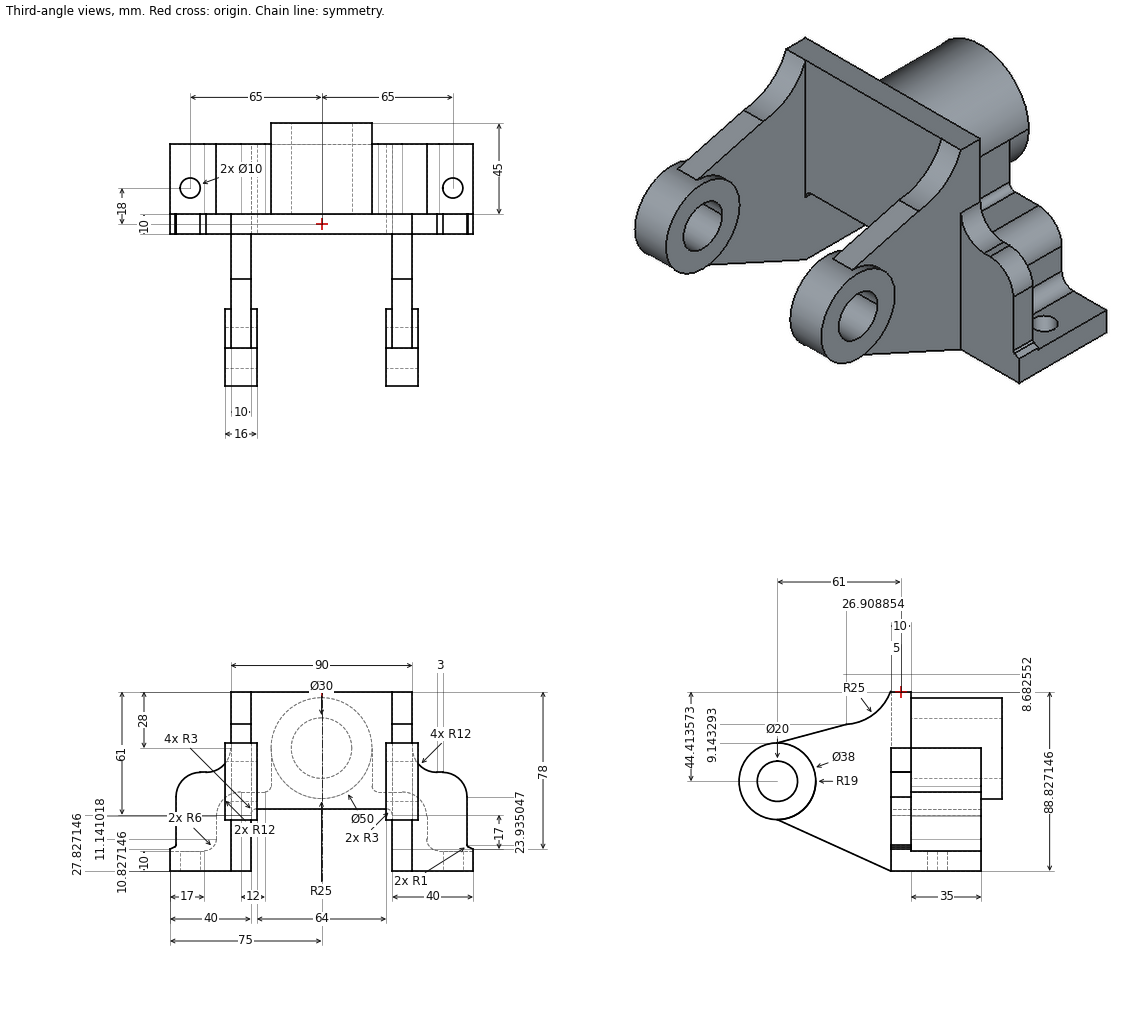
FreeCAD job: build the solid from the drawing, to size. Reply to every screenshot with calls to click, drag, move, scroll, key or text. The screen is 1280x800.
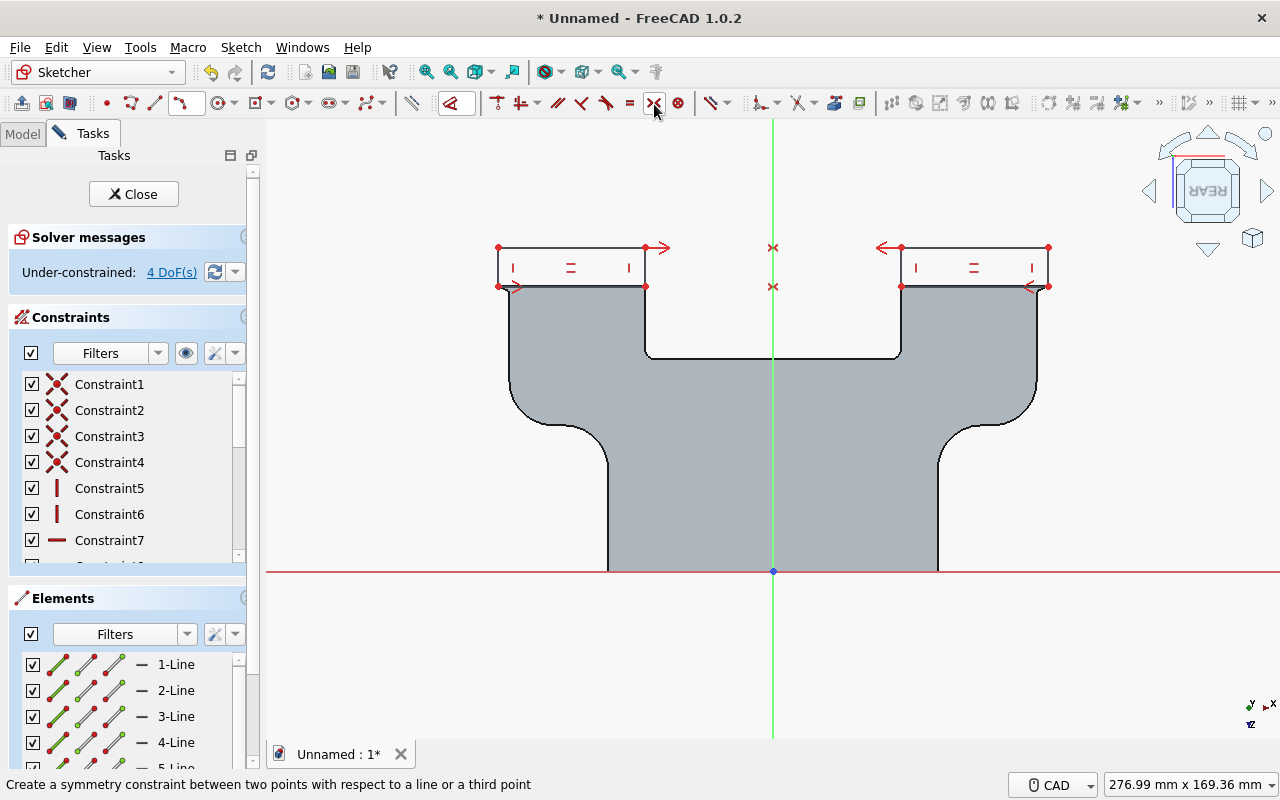
key(d)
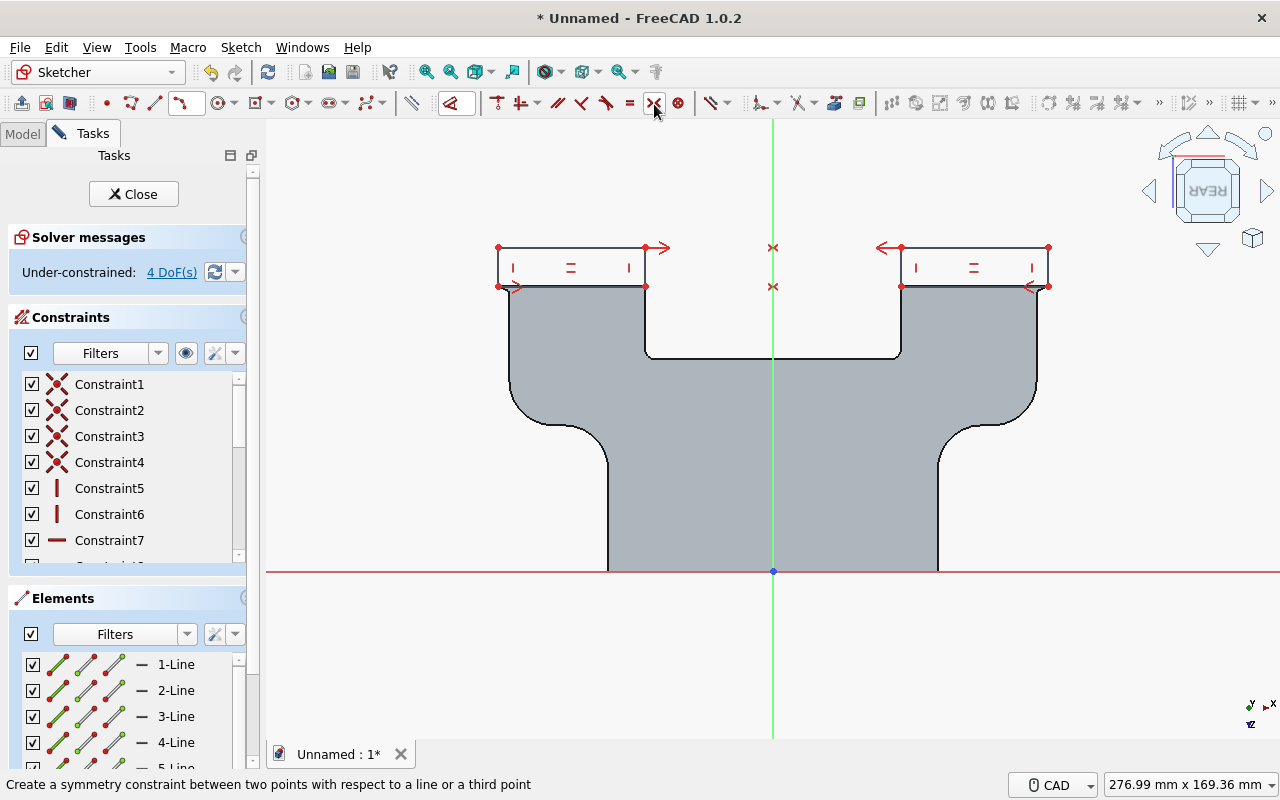
click(542, 287)
click(572, 321)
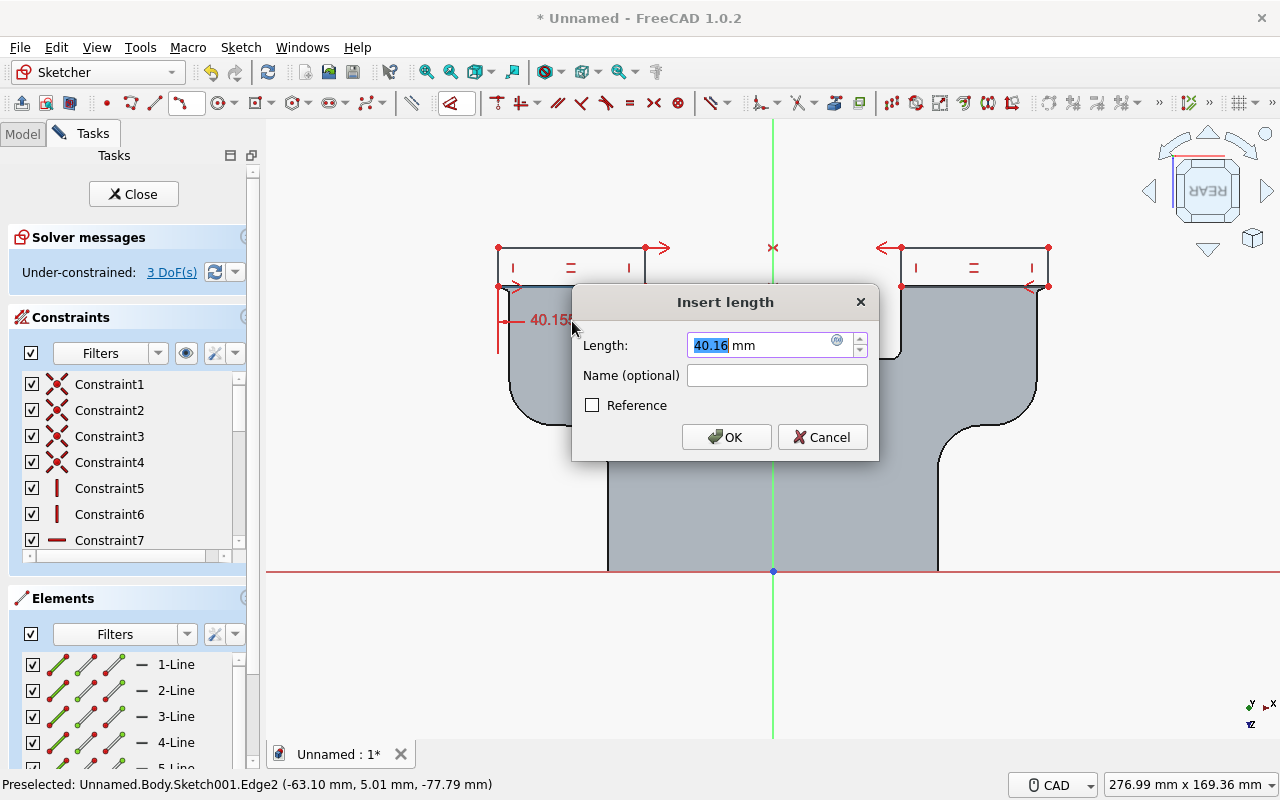
text(40)
key(Return)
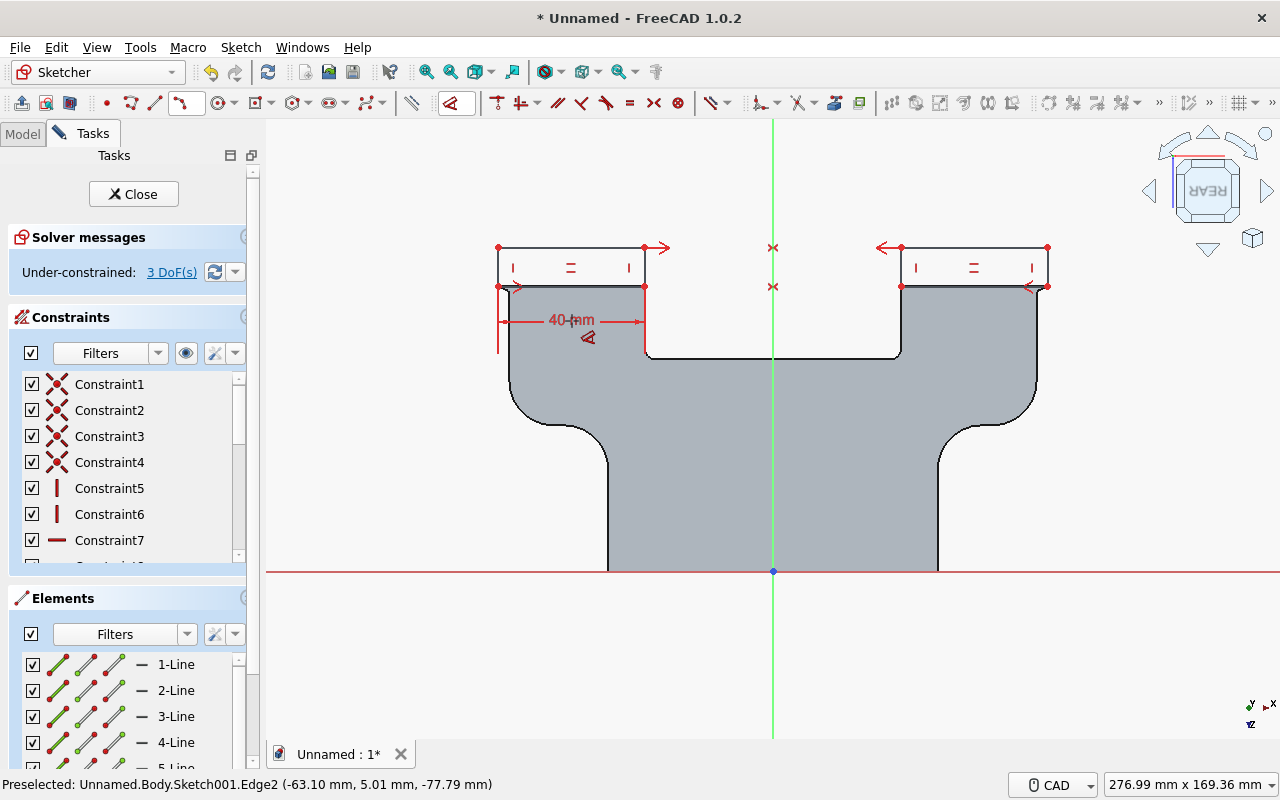
click(498, 248)
click(636, 606)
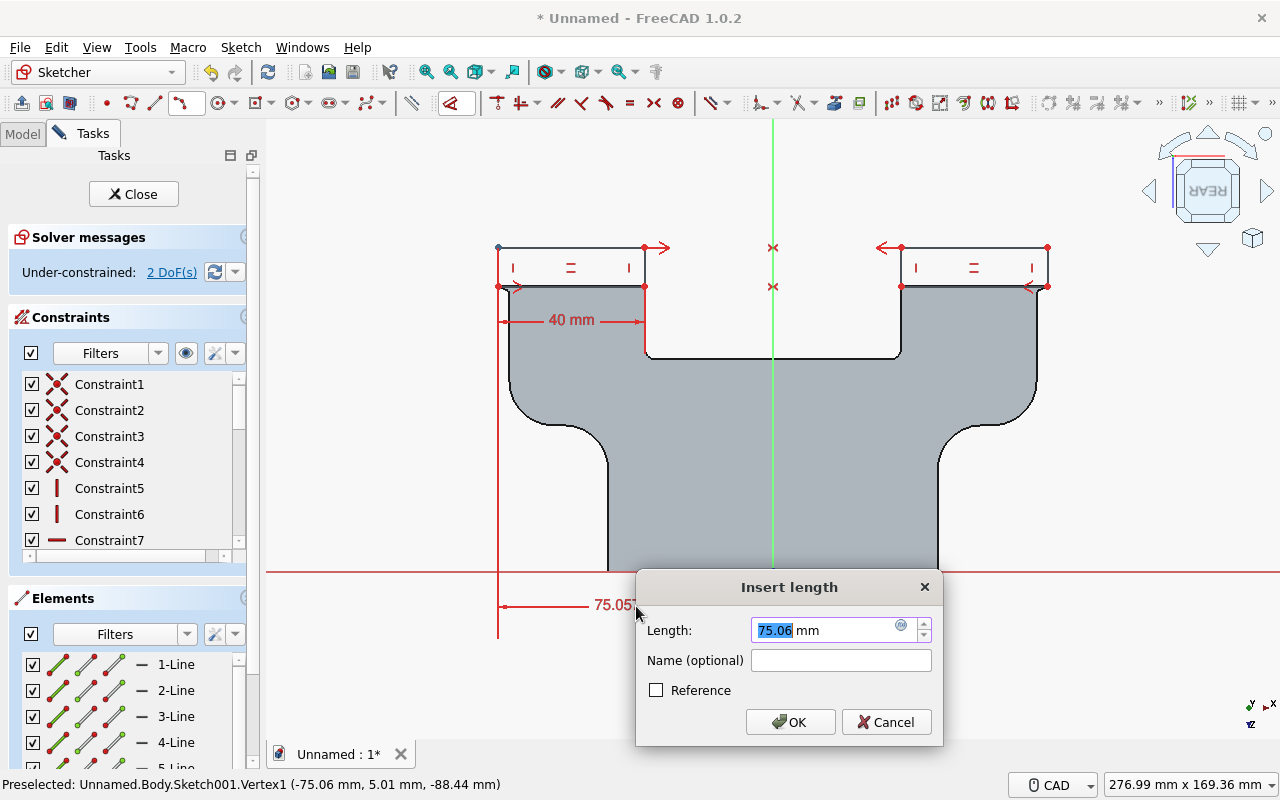
text(75)
key(Return)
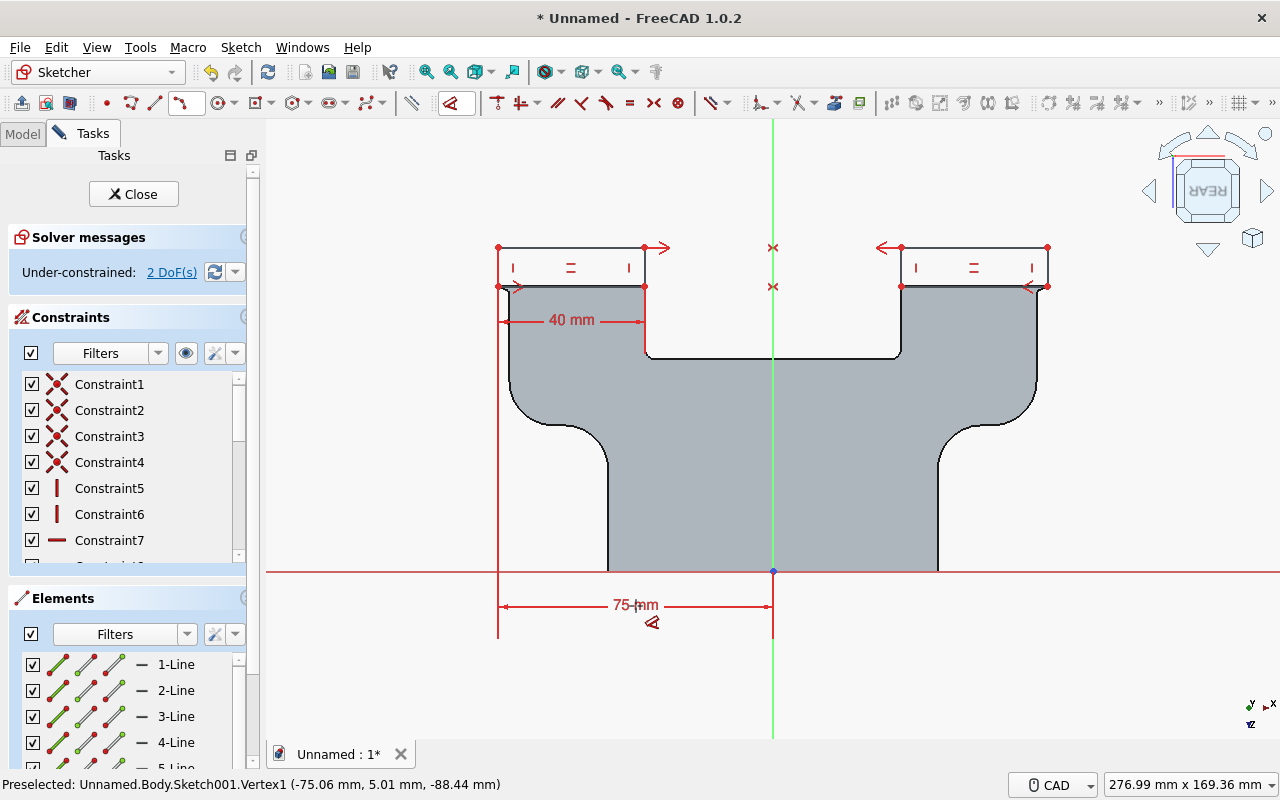
click(498, 287)
click(464, 429)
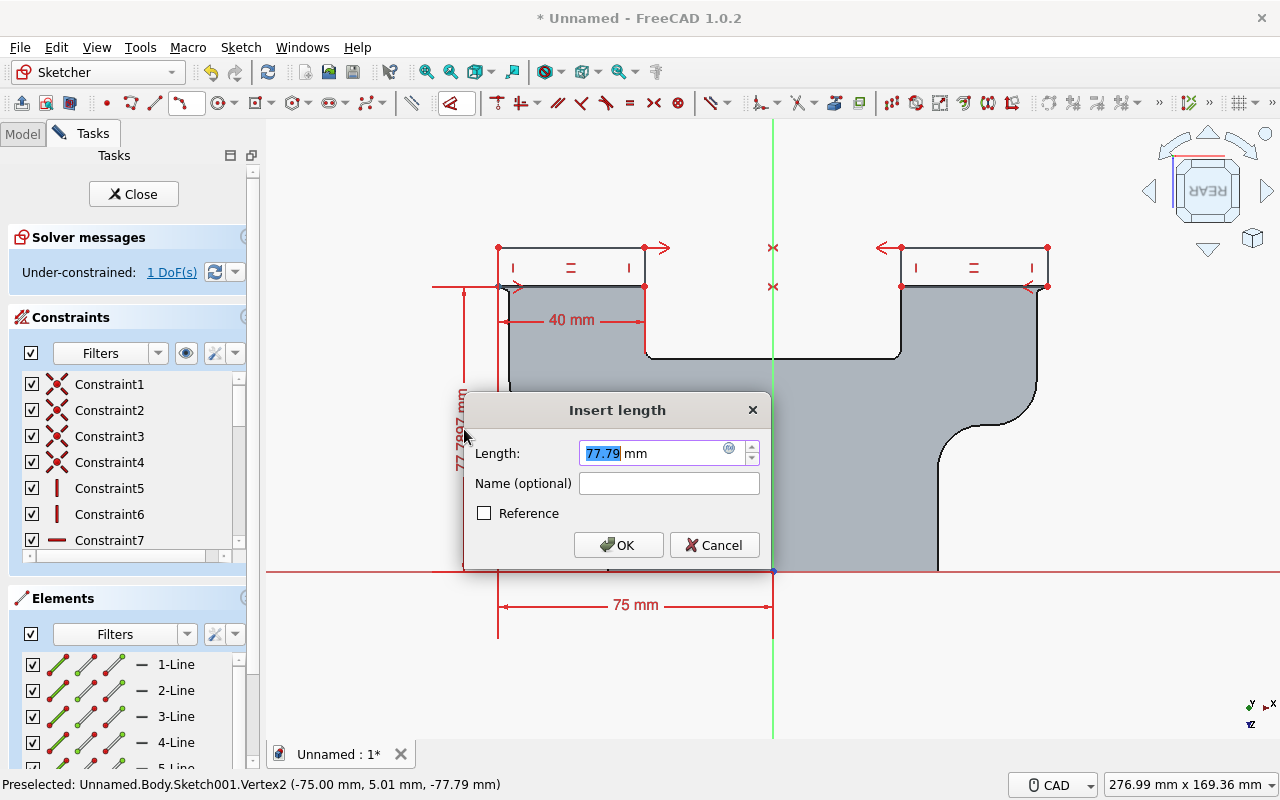
text(78)
key(Return)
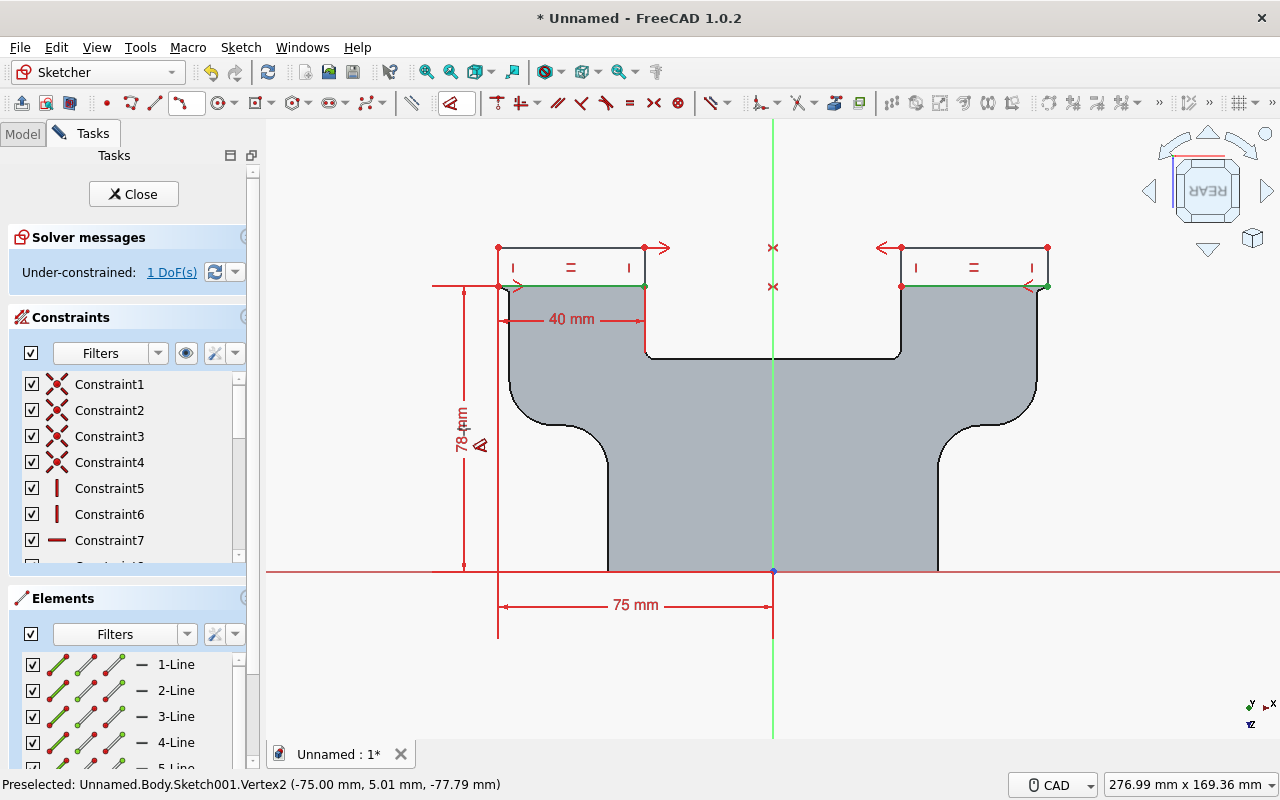
click(498, 259)
click(464, 267)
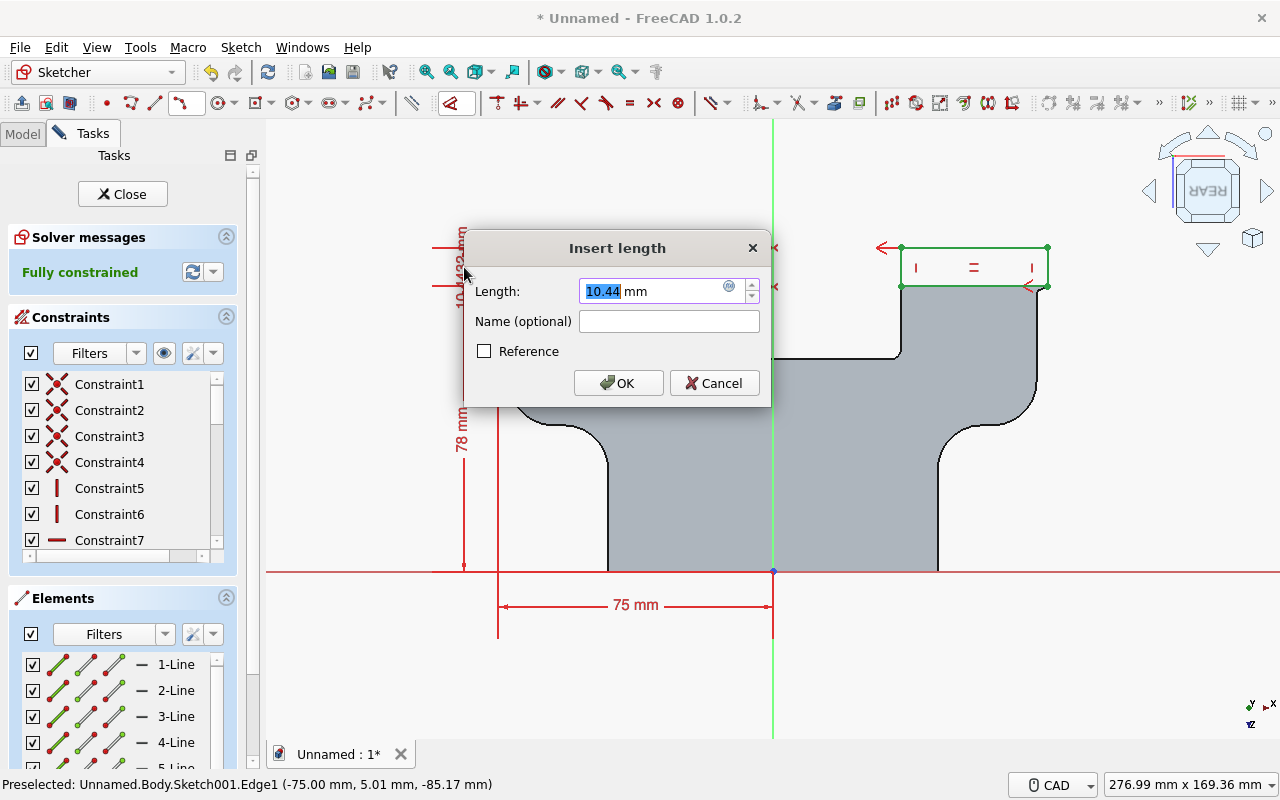
text(10.827146)
key(Return)
key(Escape)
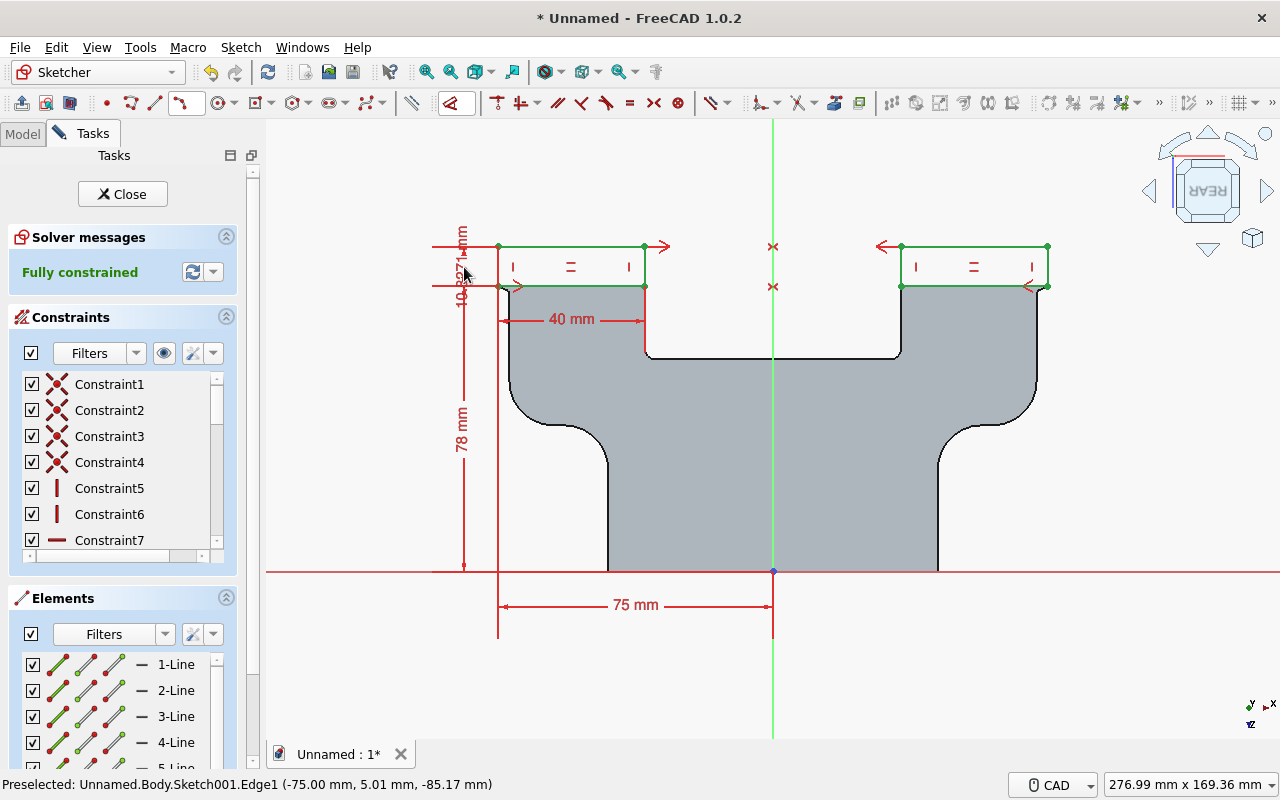
click(123, 194)